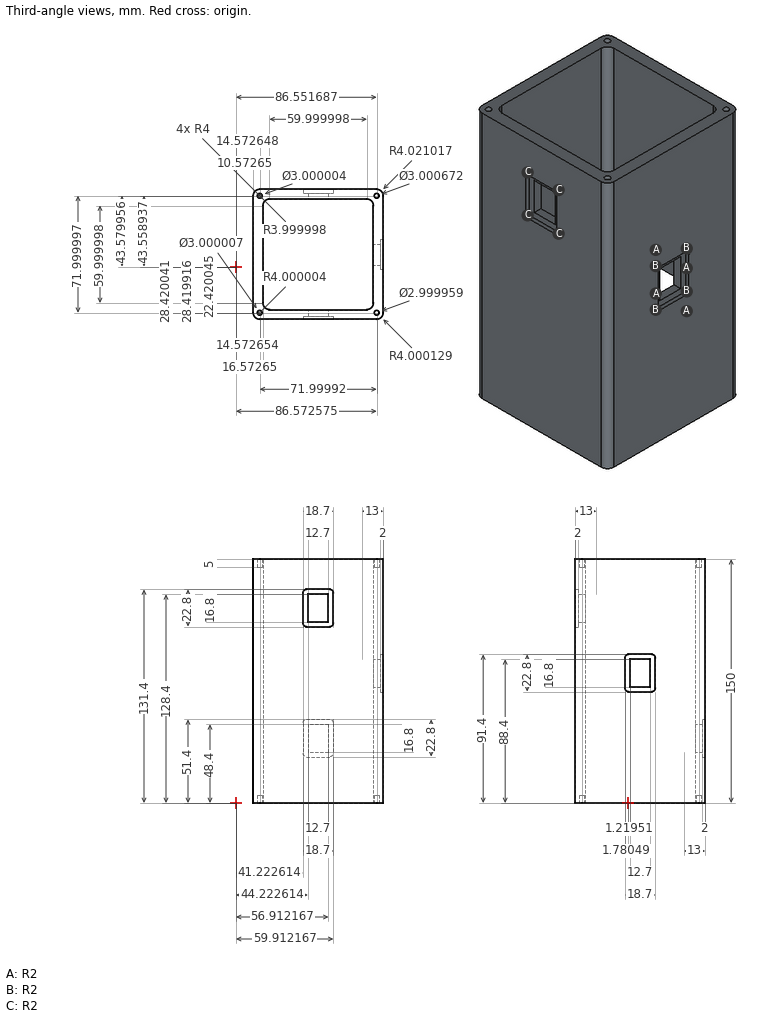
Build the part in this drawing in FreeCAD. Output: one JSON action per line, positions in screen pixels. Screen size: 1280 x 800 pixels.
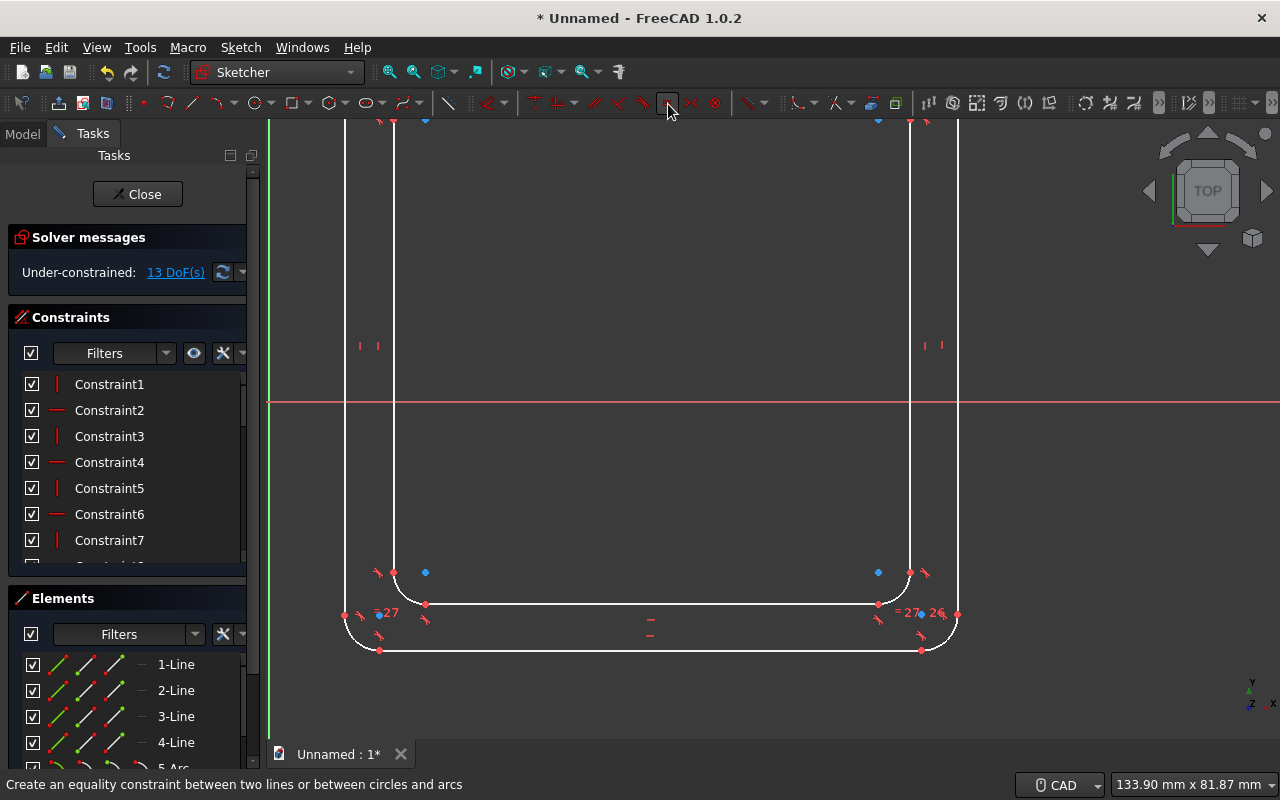
{"action": "left_click", "coordinate": [488, 104]}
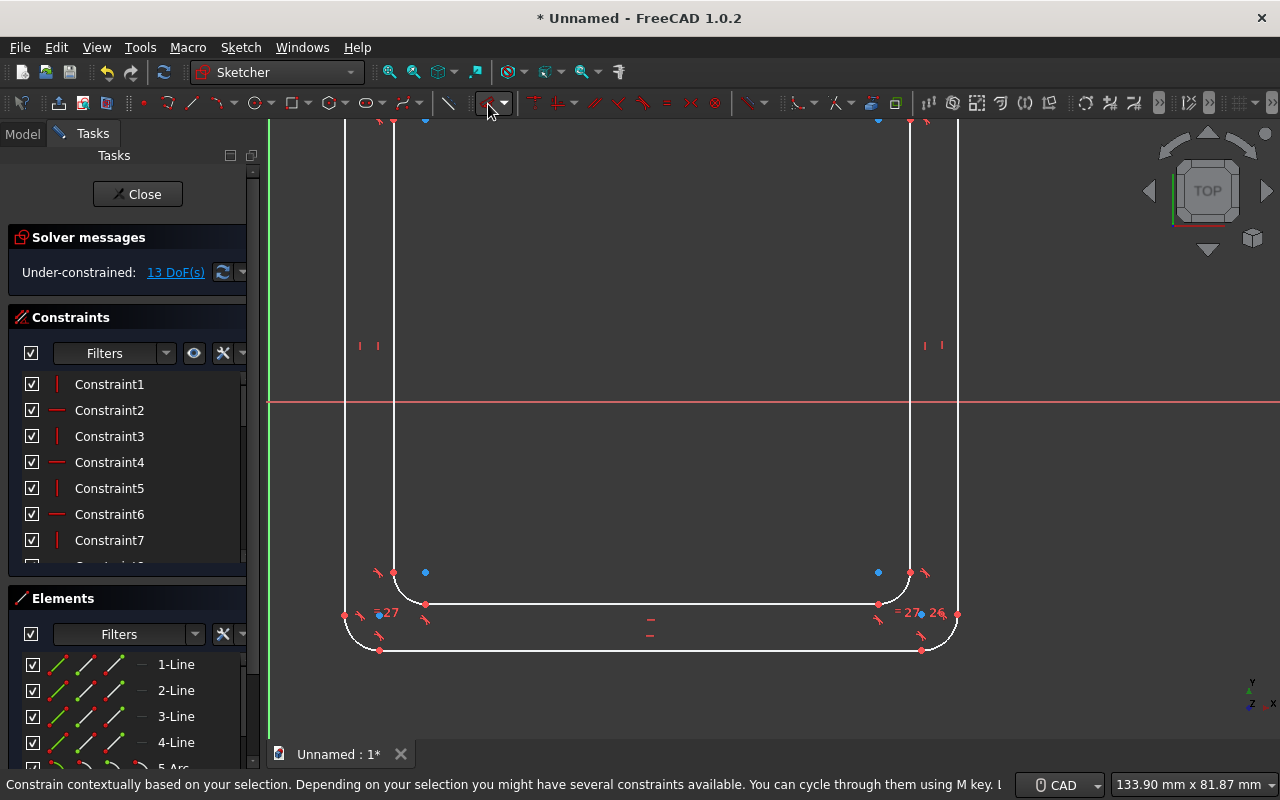
{"action": "scroll", "coordinate": [349, 632], "scroll_direction": "up", "scroll_amount": 2}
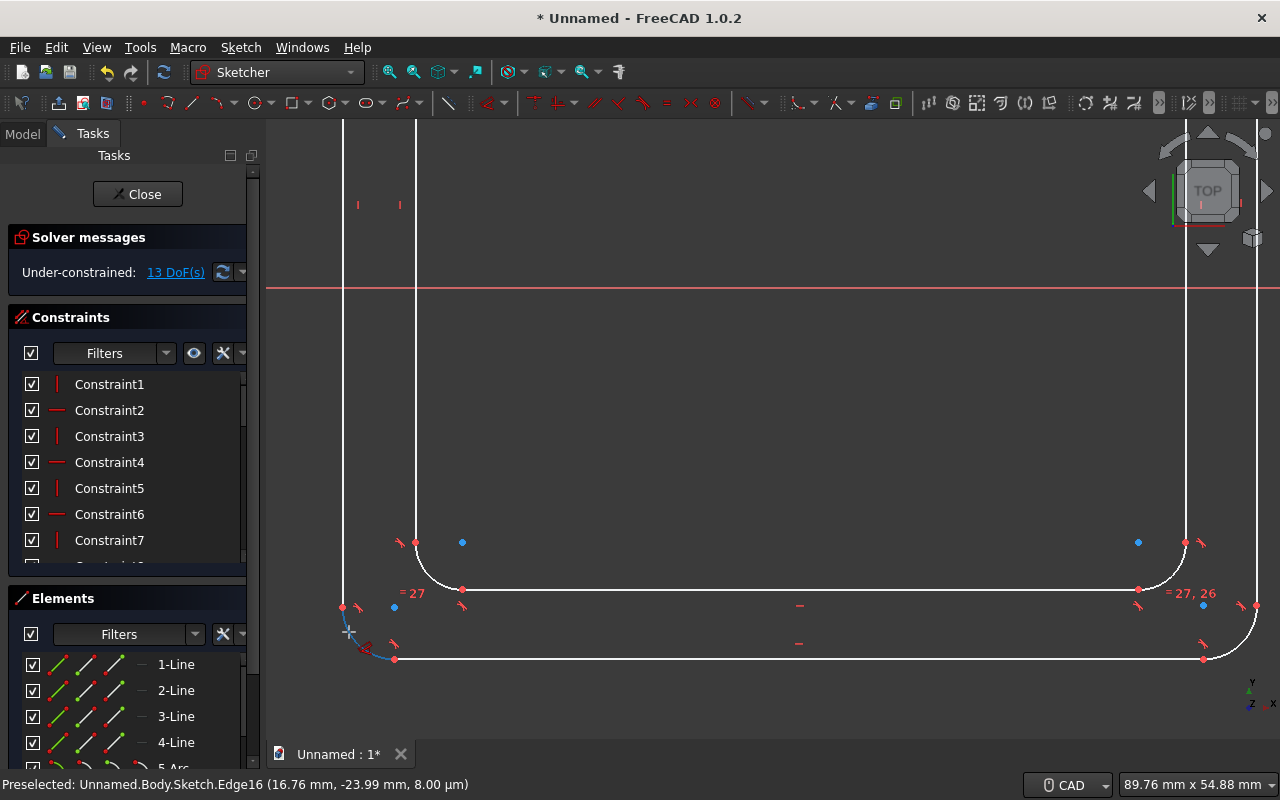
{"action": "left_click", "coordinate": [348, 631]}
{"action": "left_click", "coordinate": [319, 645]}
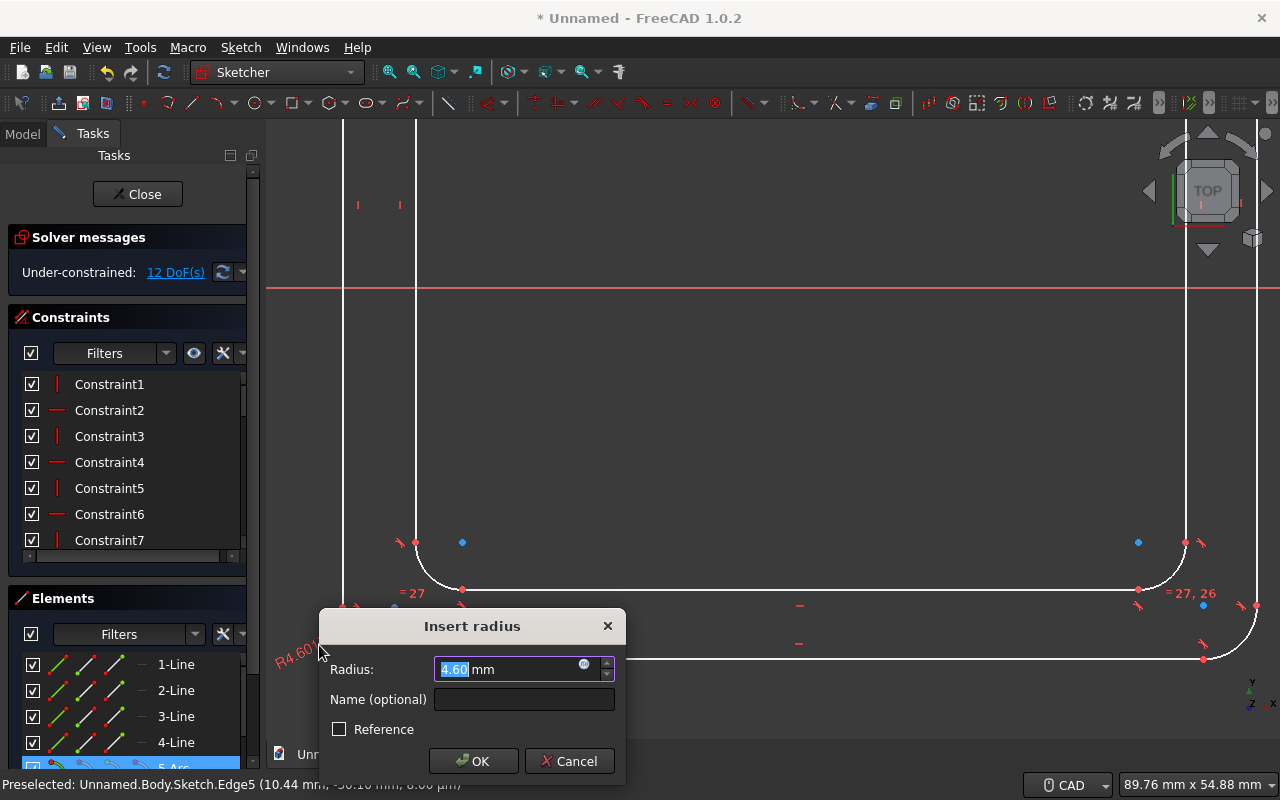
{"action": "type", "text": "4.000004"}
{"action": "key", "text": "Return"}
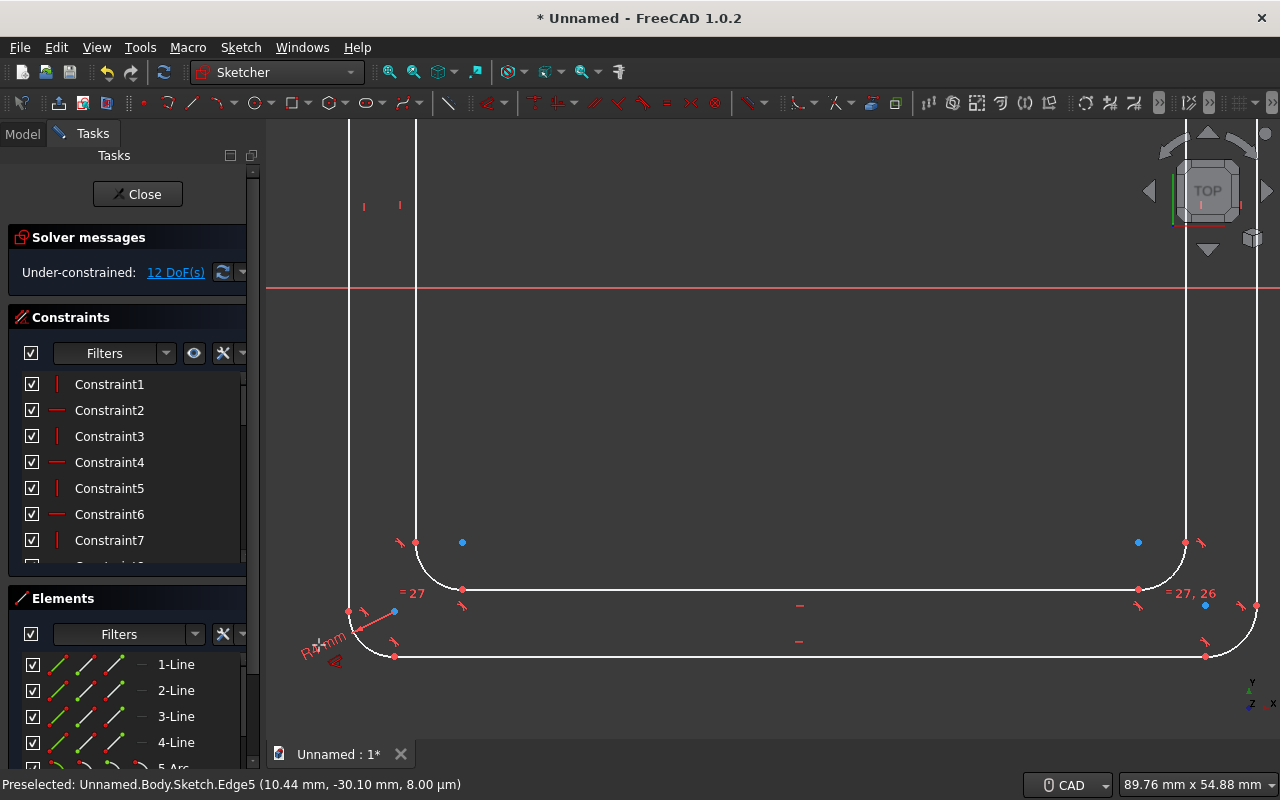
{"action": "scroll", "coordinate": [675, 614], "scroll_direction": "down", "scroll_amount": 4}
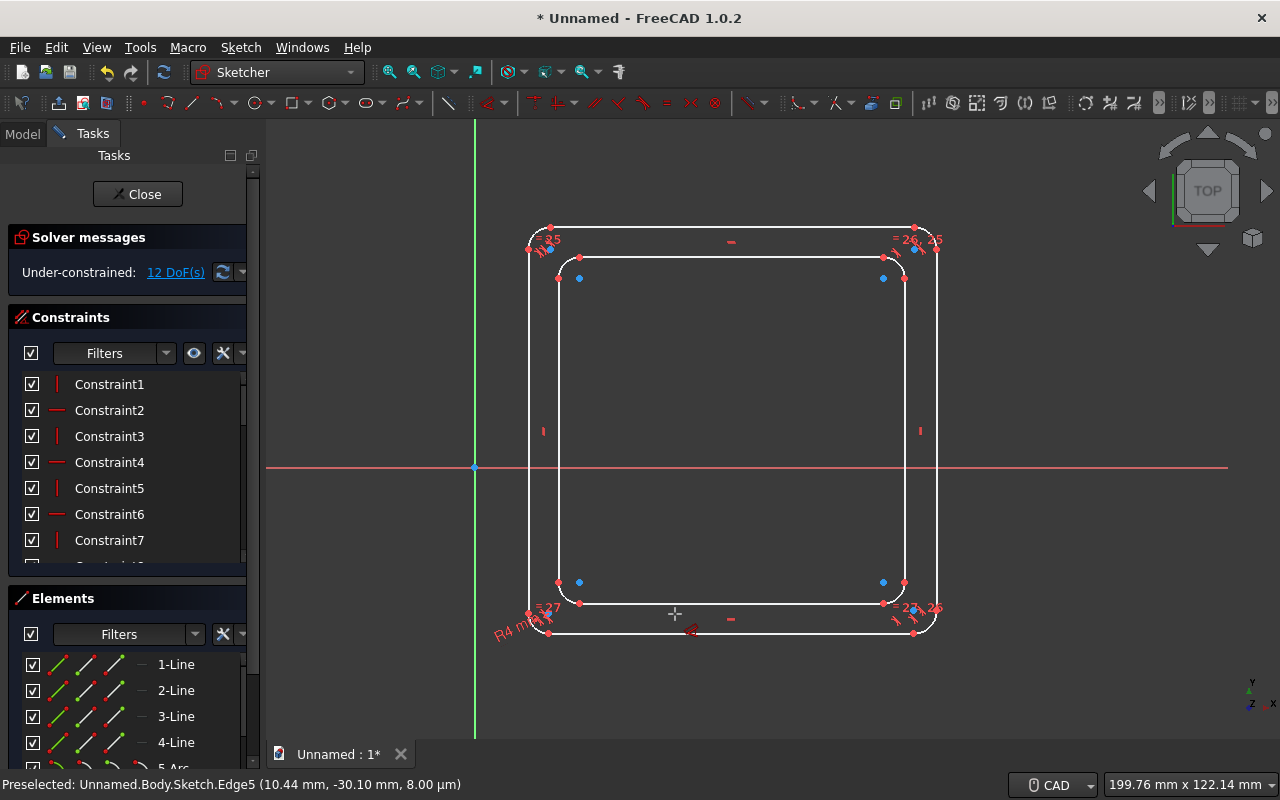
{"action": "scroll", "coordinate": [924, 631], "scroll_direction": "up", "scroll_amount": 4}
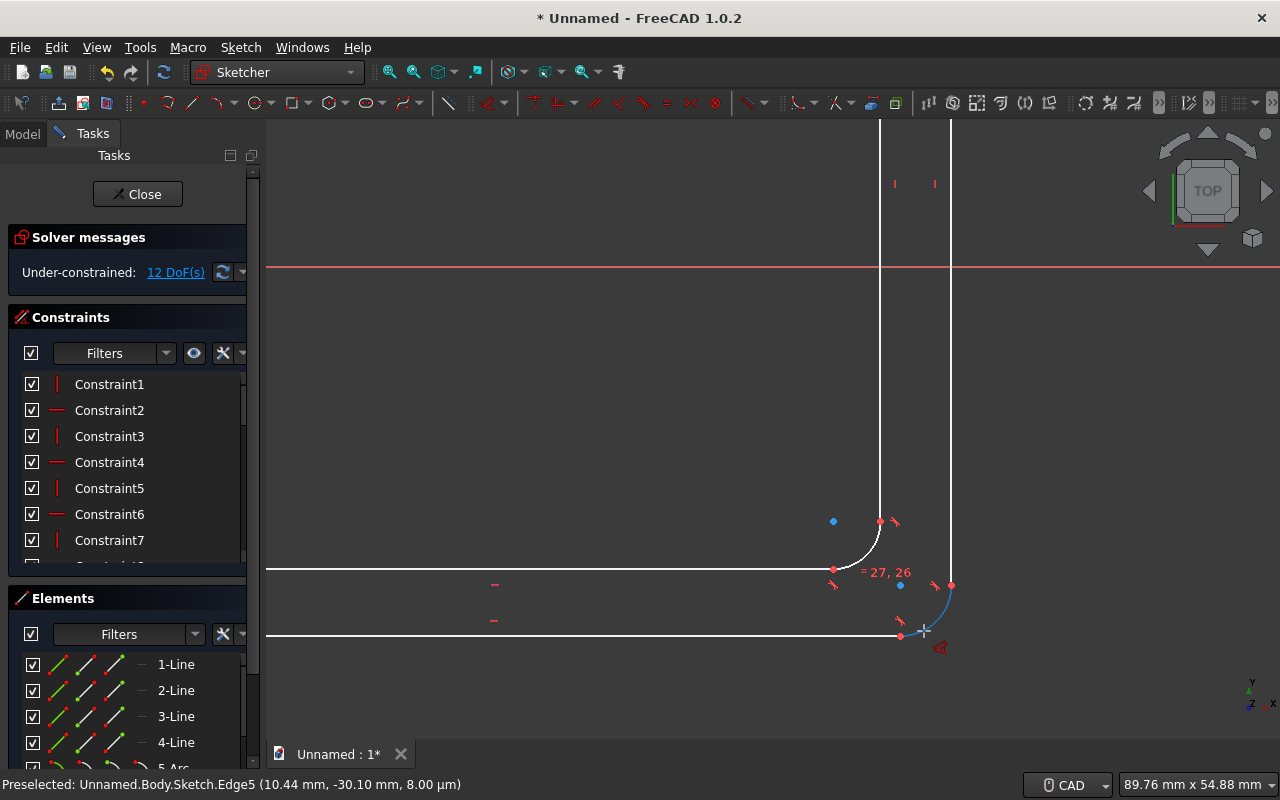
{"action": "left_click", "coordinate": [924, 631]}
{"action": "left_click", "coordinate": [939, 659]}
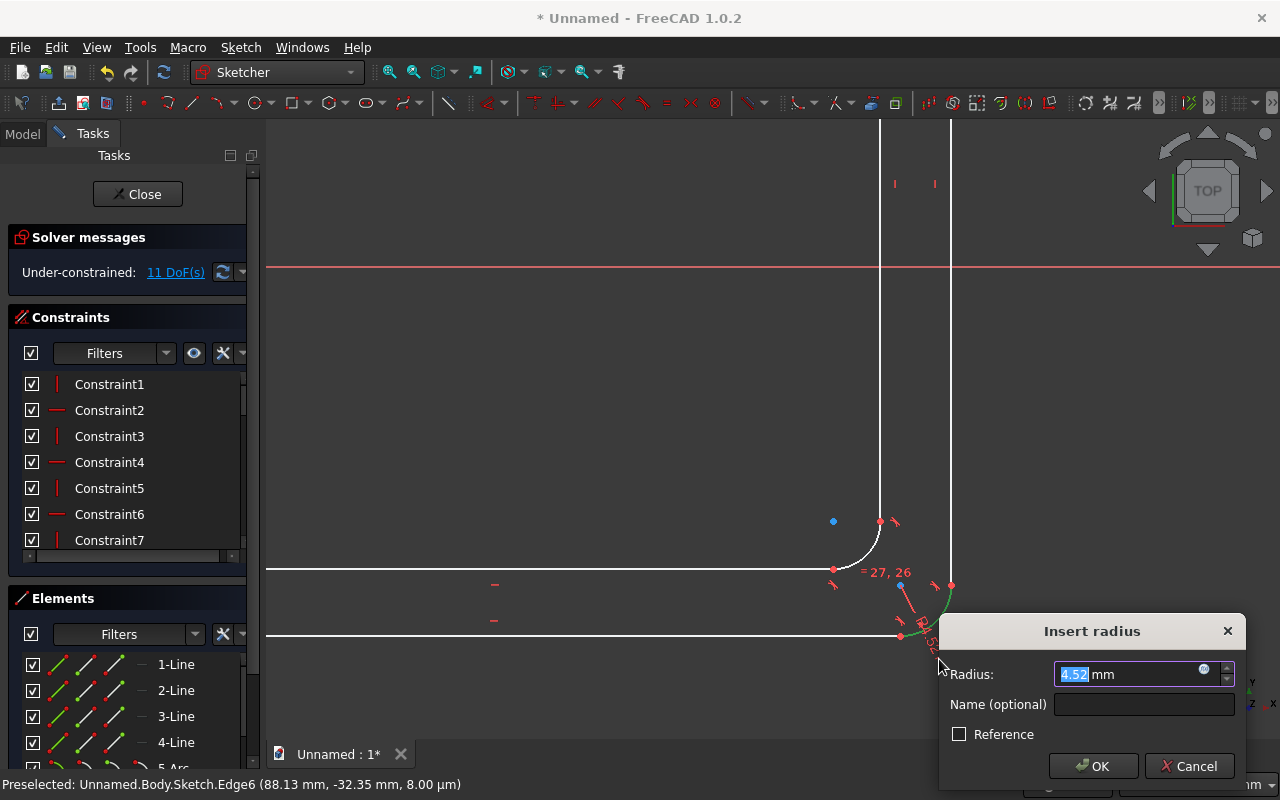
{"action": "type", "text": "4.000129"}
{"action": "key", "text": "Return"}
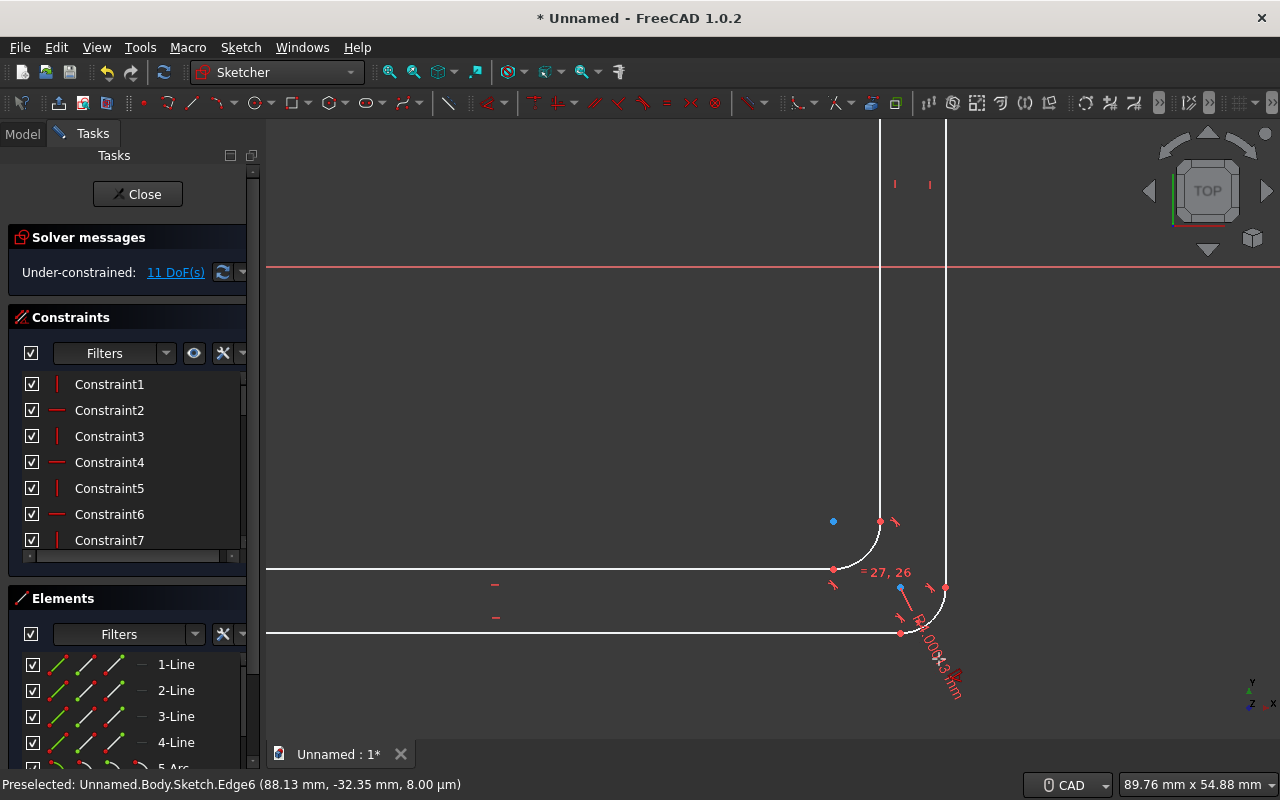
{"action": "scroll", "coordinate": [924, 631], "scroll_direction": "down", "scroll_amount": 4}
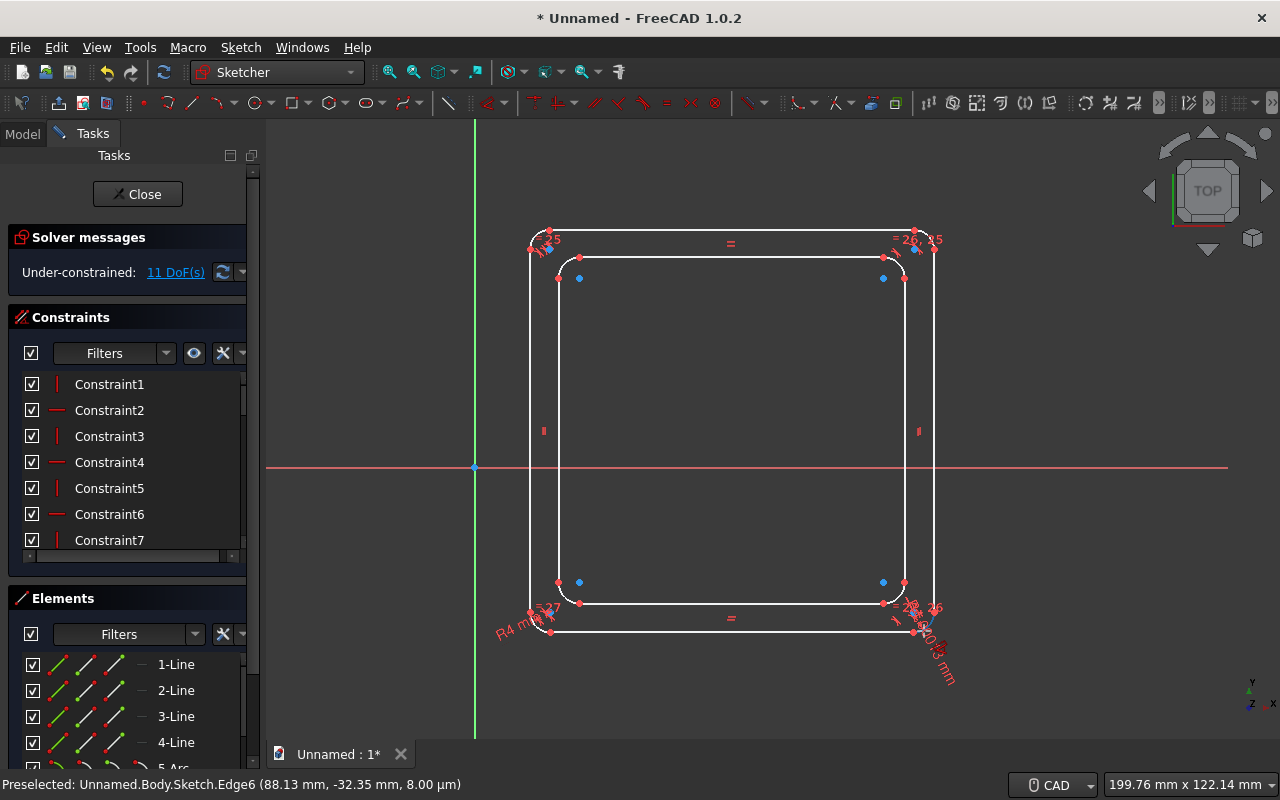
{"action": "scroll", "coordinate": [932, 241], "scroll_direction": "up", "scroll_amount": 4}